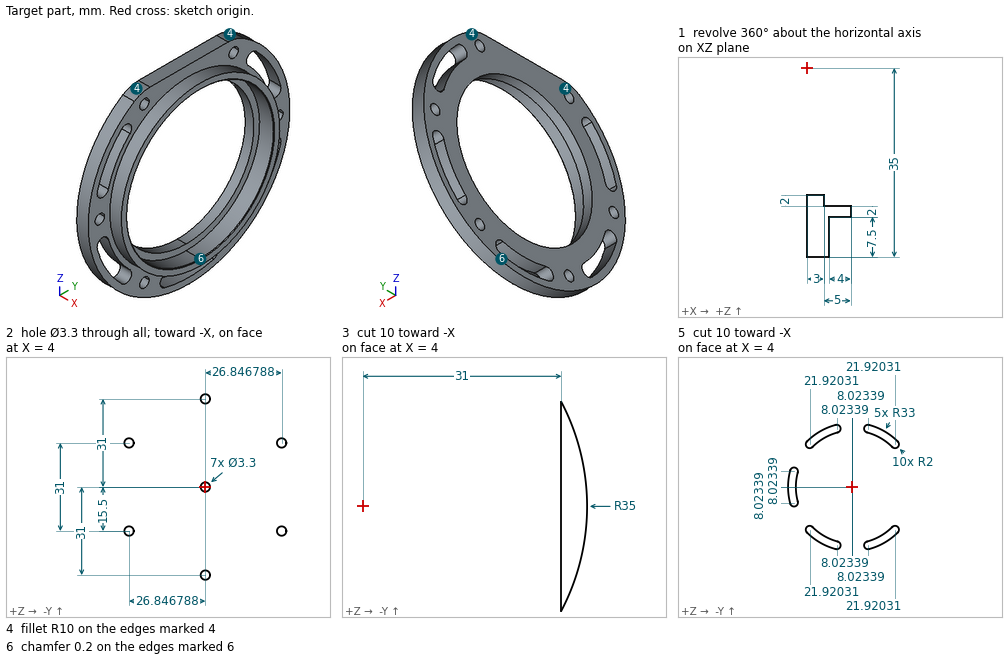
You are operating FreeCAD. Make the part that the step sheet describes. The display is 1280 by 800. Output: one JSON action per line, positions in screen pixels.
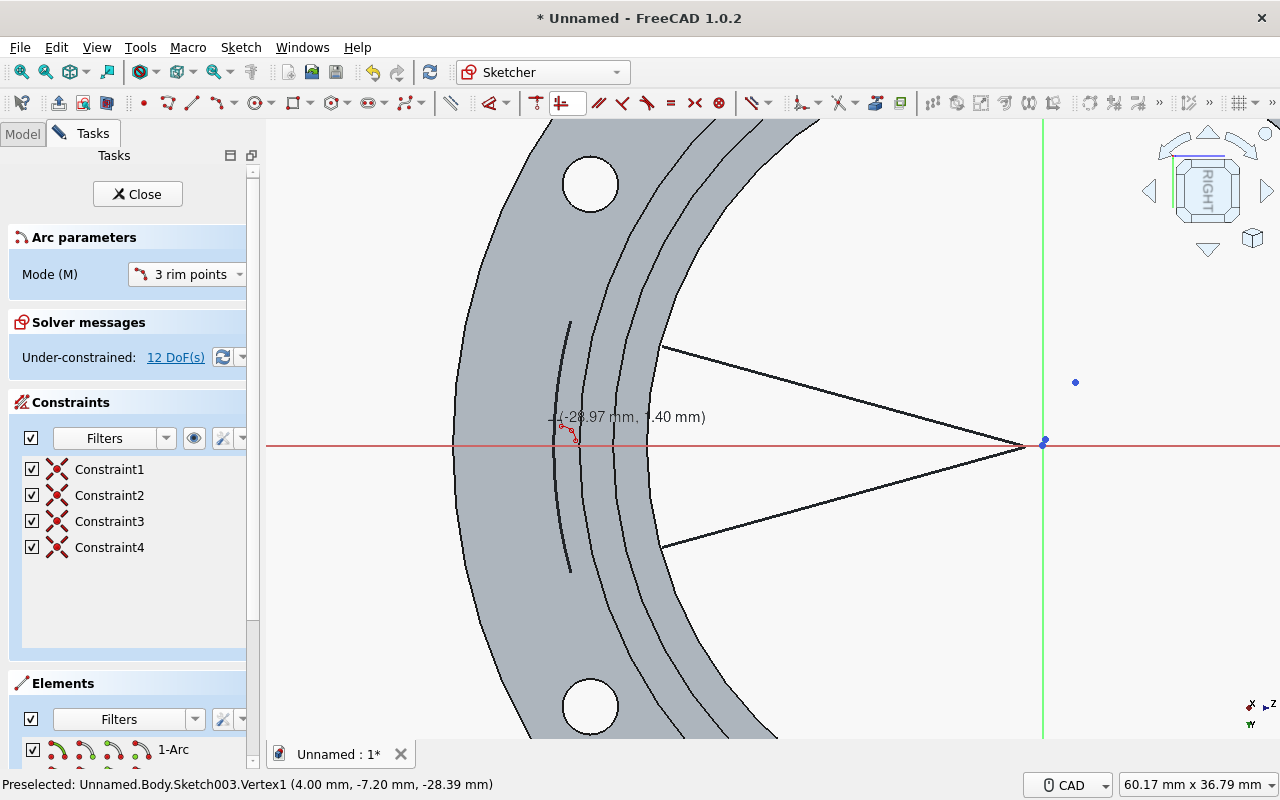
{"action": "left_click", "coordinate": [555, 420]}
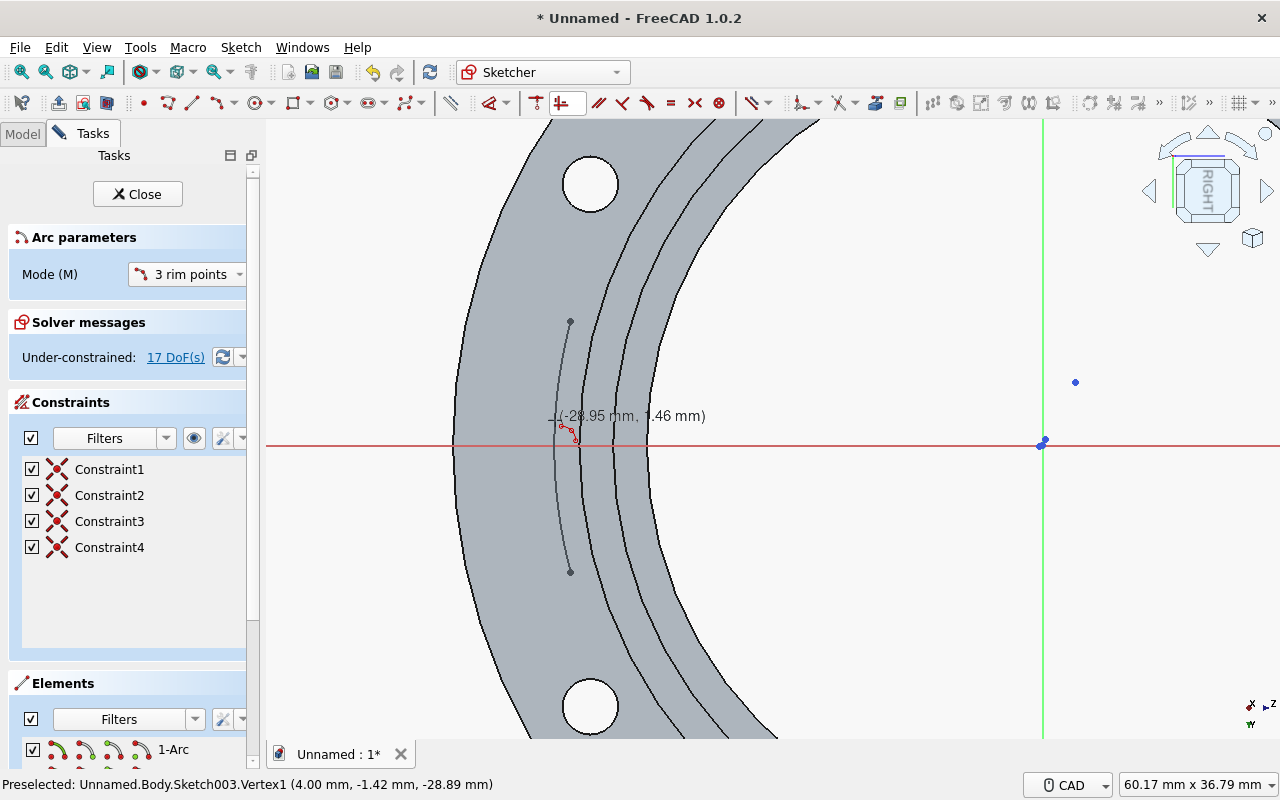
{"action": "left_click", "coordinate": [571, 321]}
{"action": "left_click", "coordinate": [506, 302]}
{"action": "left_click", "coordinate": [547, 278]}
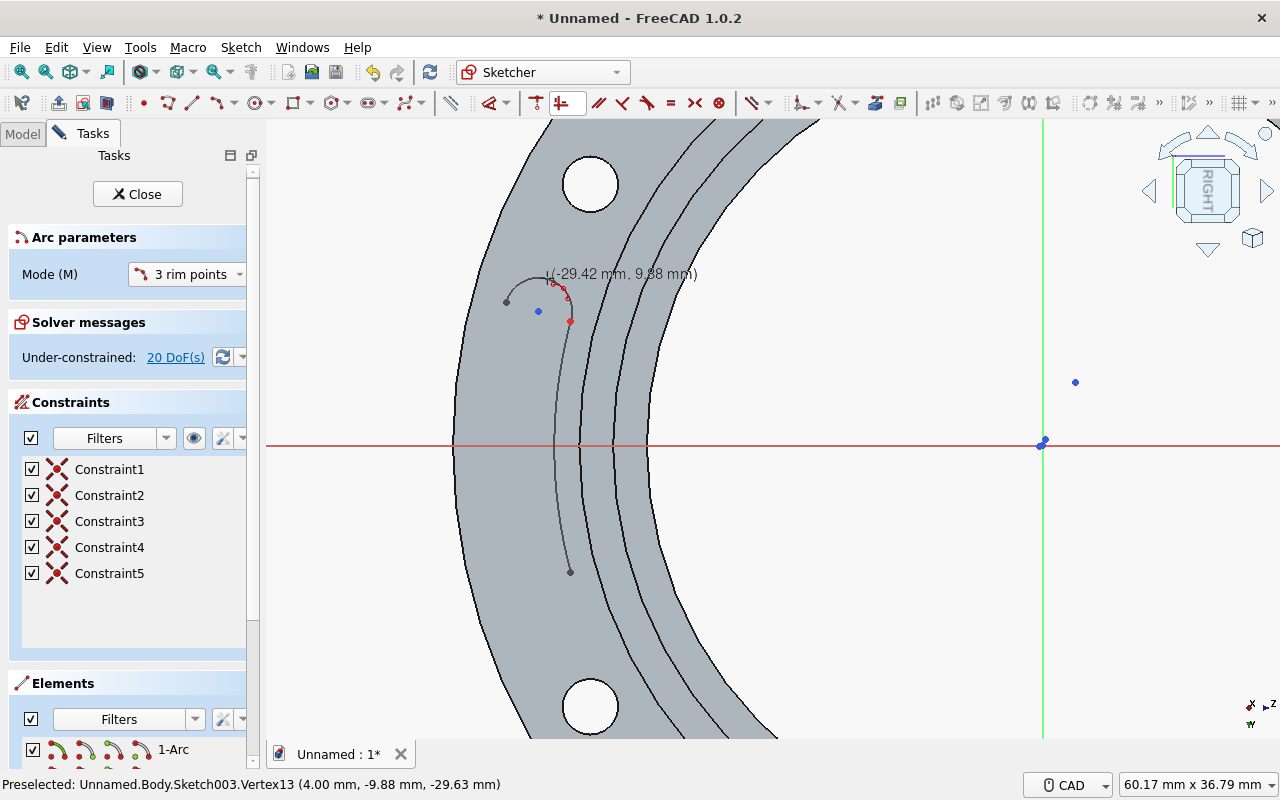
{"action": "left_click", "coordinate": [506, 303]}
{"action": "left_click", "coordinate": [506, 589]}
{"action": "left_click", "coordinate": [487, 416]}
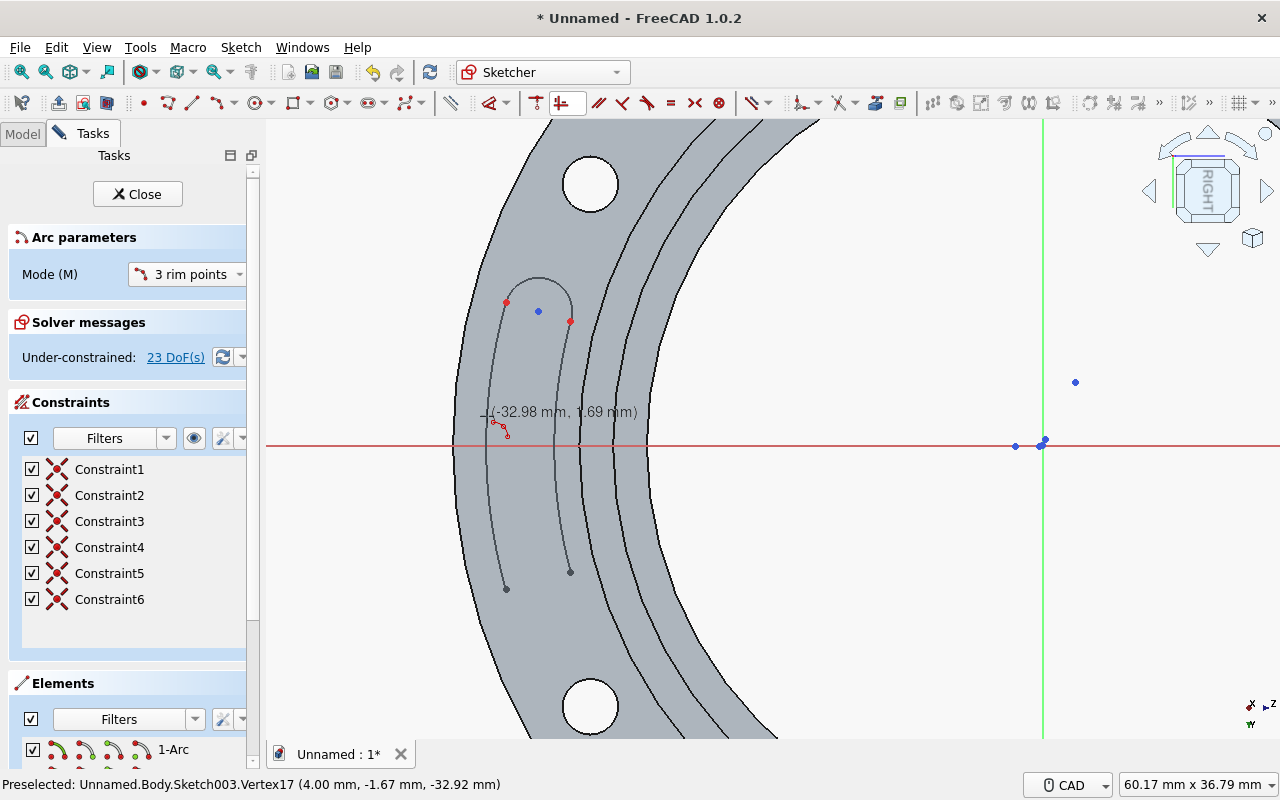
{"action": "left_click", "coordinate": [506, 590]}
{"action": "left_click", "coordinate": [571, 573]}
{"action": "left_click", "coordinate": [547, 613]}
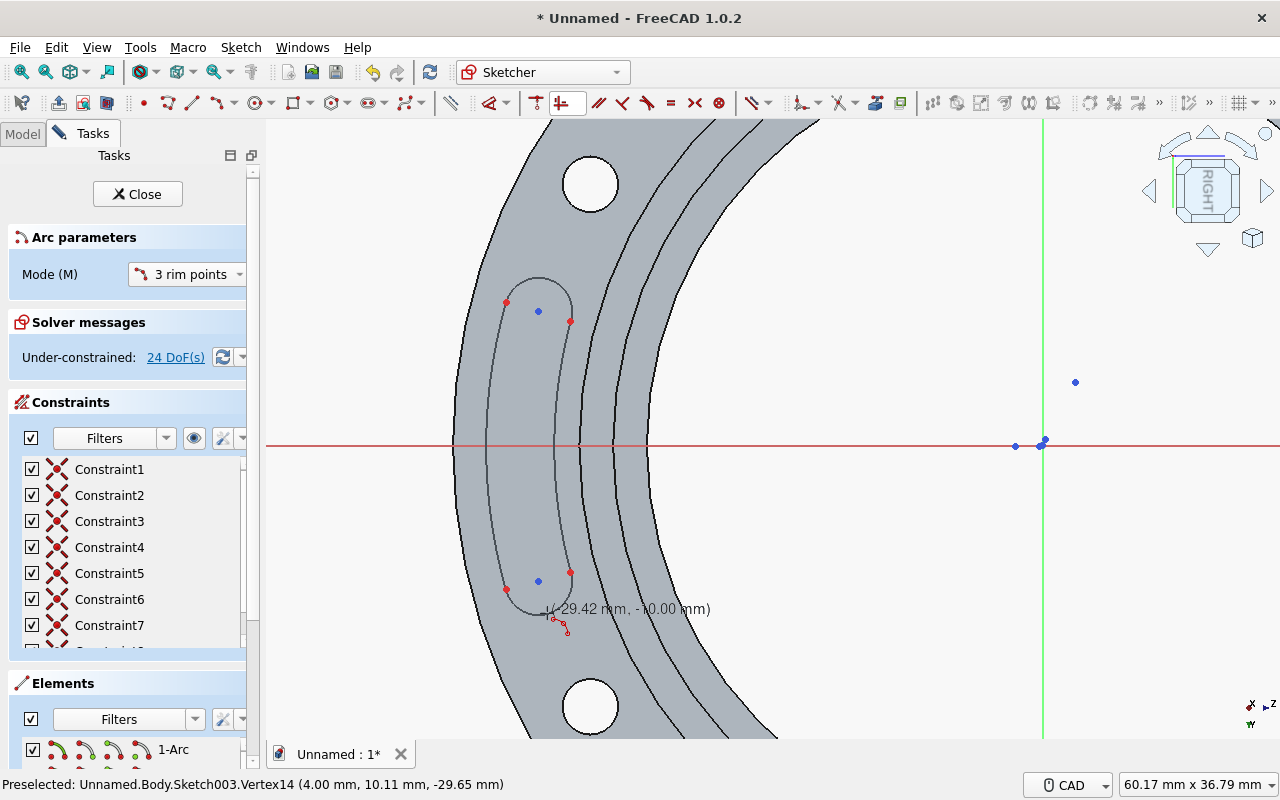
{"action": "scroll", "coordinate": [555, 419], "scroll_direction": "down", "scroll_amount": 5}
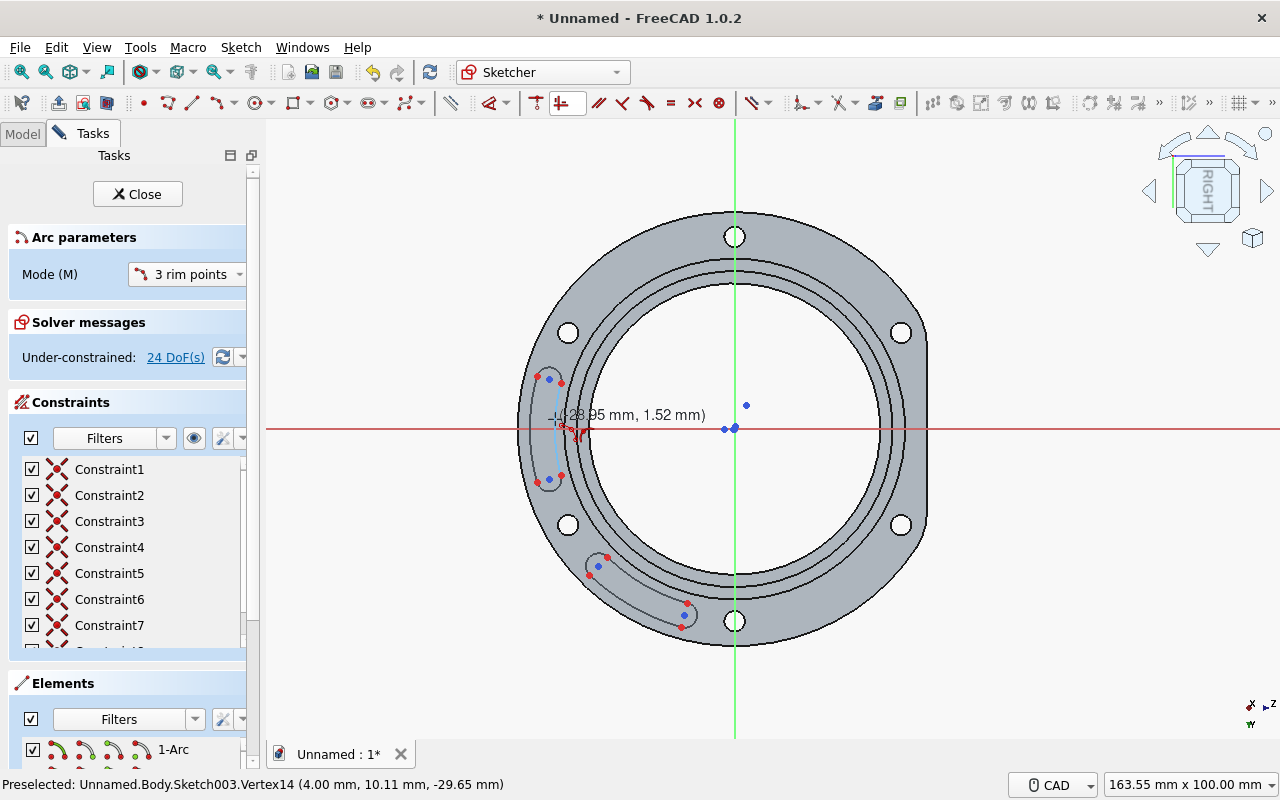
{"action": "left_click", "coordinate": [608, 302]}
{"action": "left_click", "coordinate": [688, 255]}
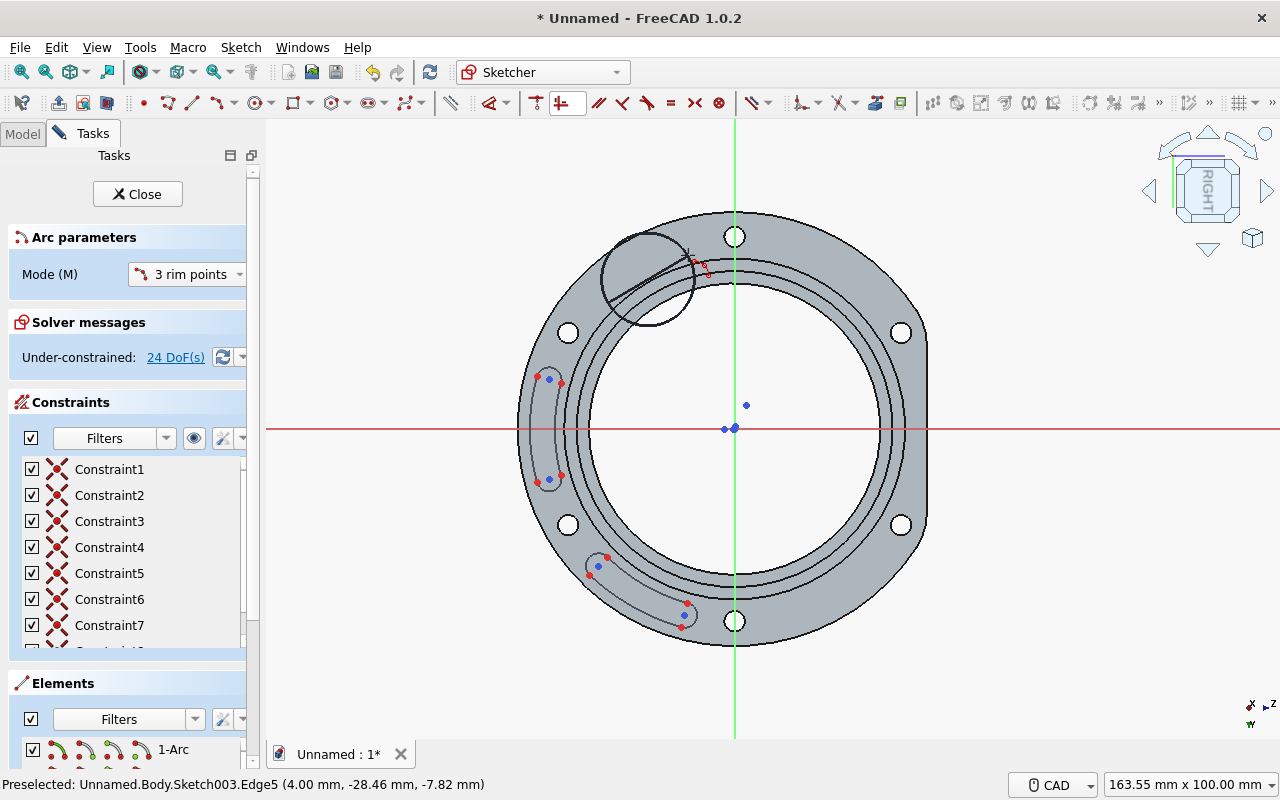
{"action": "scroll", "coordinate": [645, 273], "scroll_direction": "up", "scroll_amount": 5}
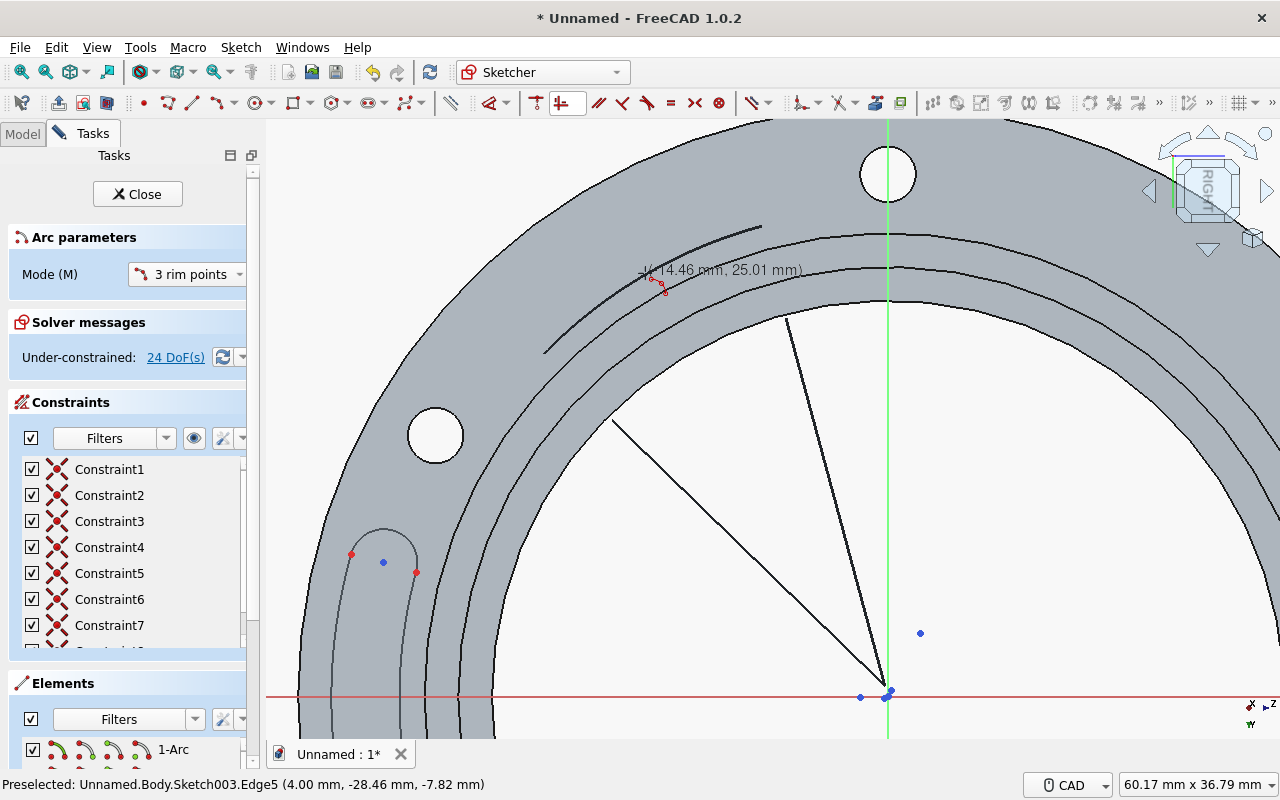
{"action": "left_click", "coordinate": [644, 274]}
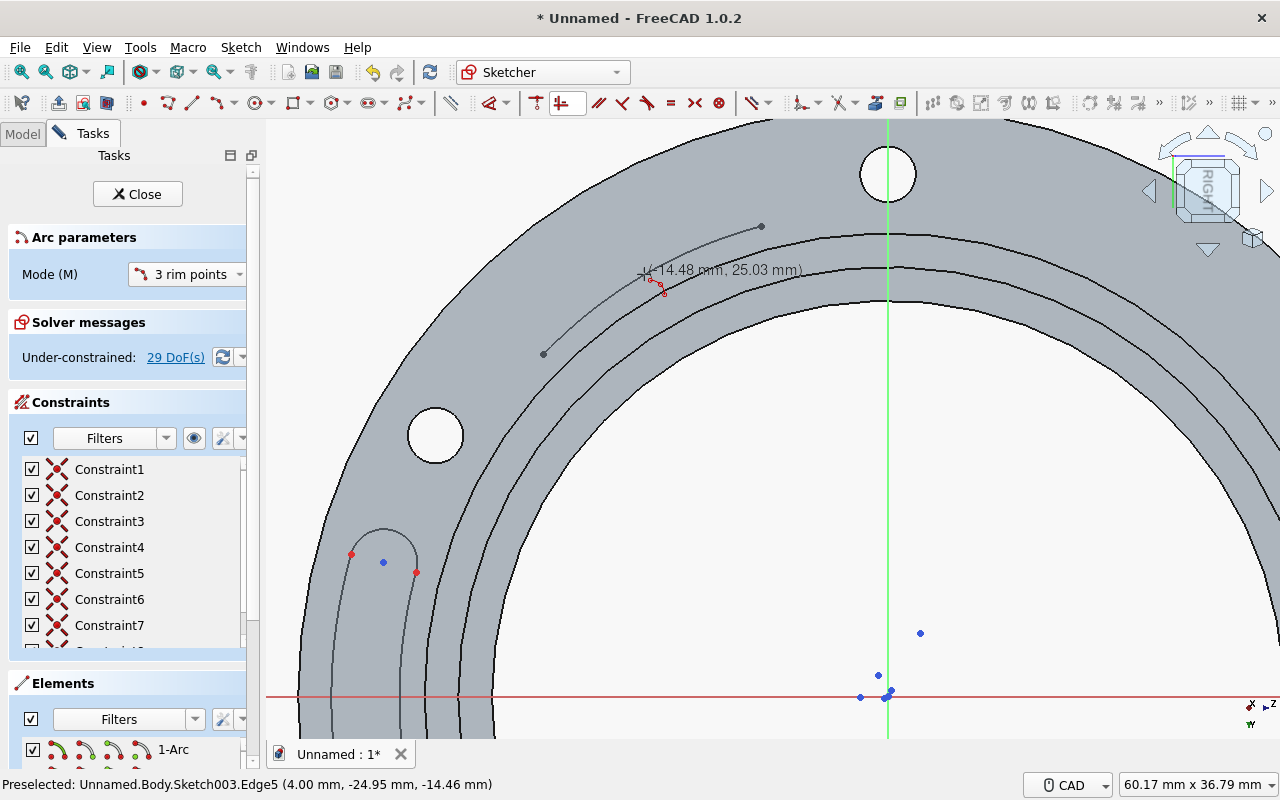
{"action": "left_click", "coordinate": [761, 226]}
{"action": "left_click", "coordinate": [744, 160]}
{"action": "left_click", "coordinate": [785, 183]}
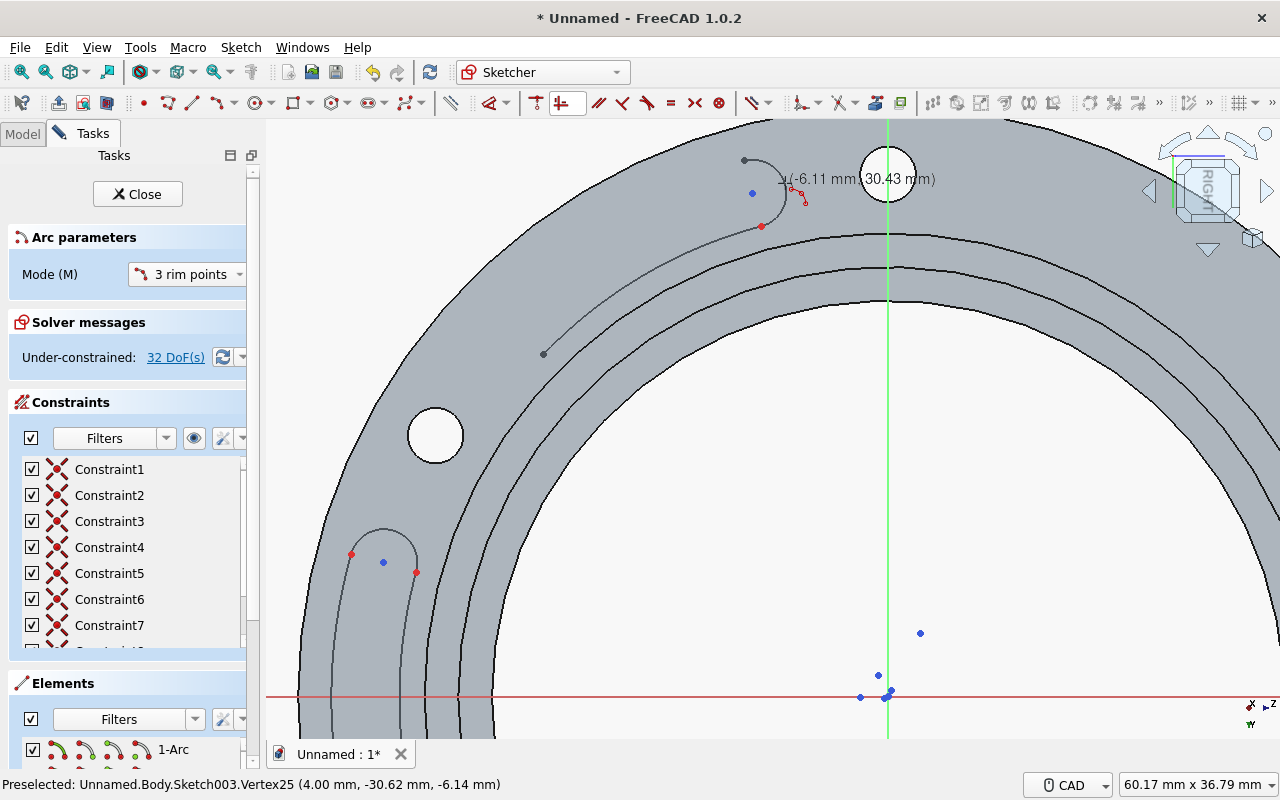
{"action": "left_click", "coordinate": [744, 161]}
{"action": "left_click", "coordinate": [495, 304]}
{"action": "left_click", "coordinate": [610, 215]}